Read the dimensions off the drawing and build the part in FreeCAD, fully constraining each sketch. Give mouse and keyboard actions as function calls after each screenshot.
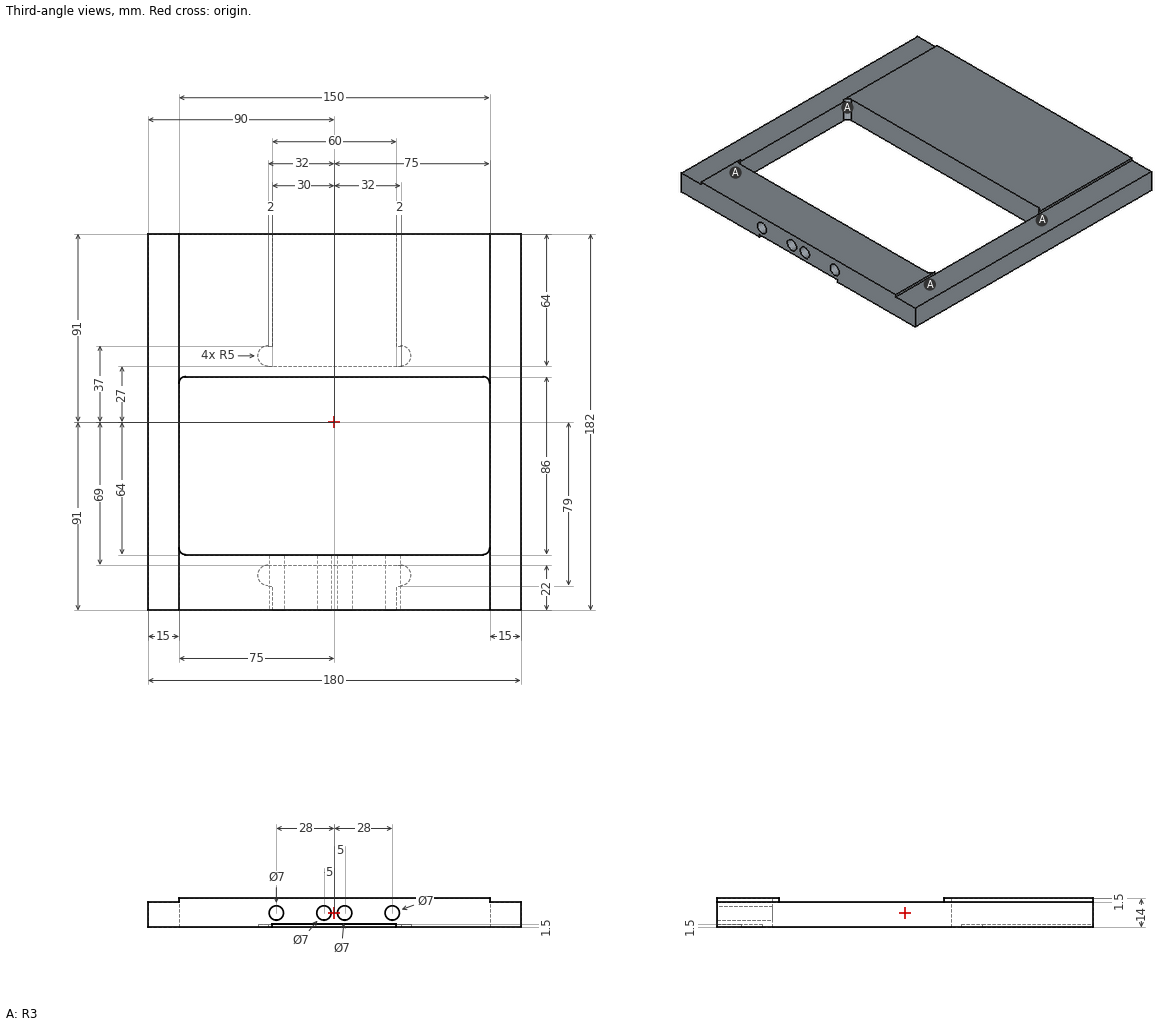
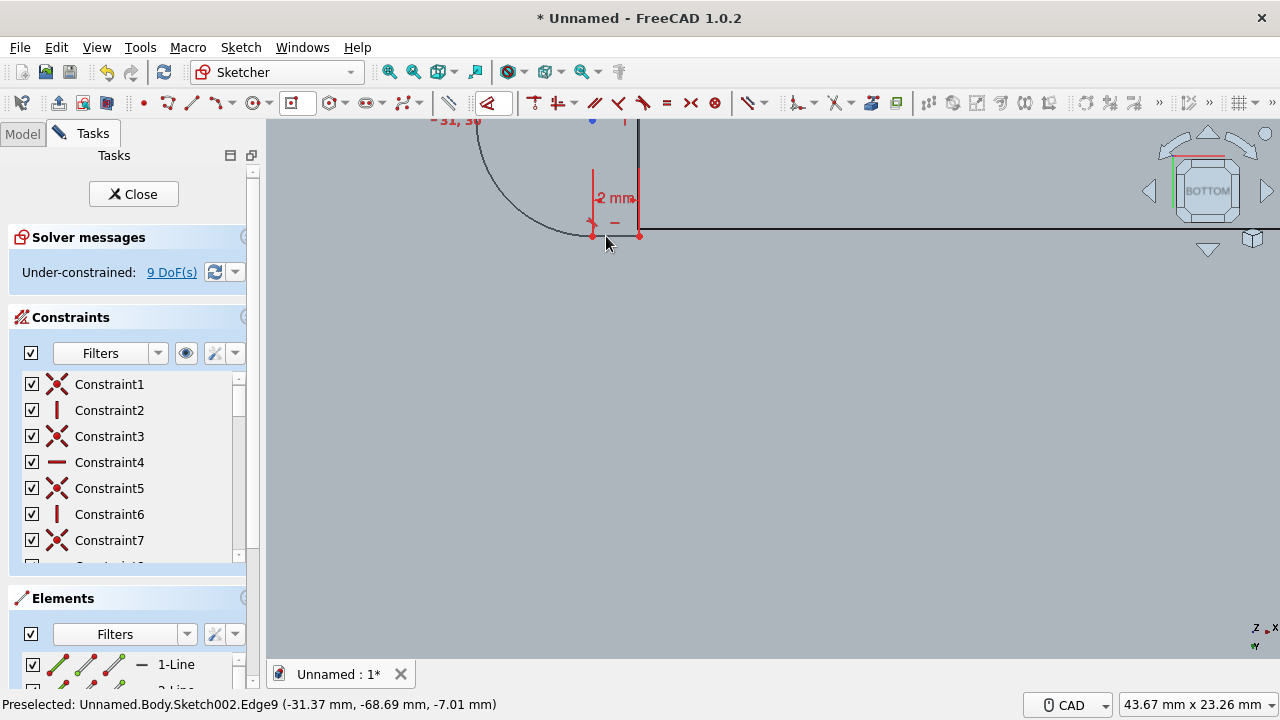
scroll(606, 240, down, 10)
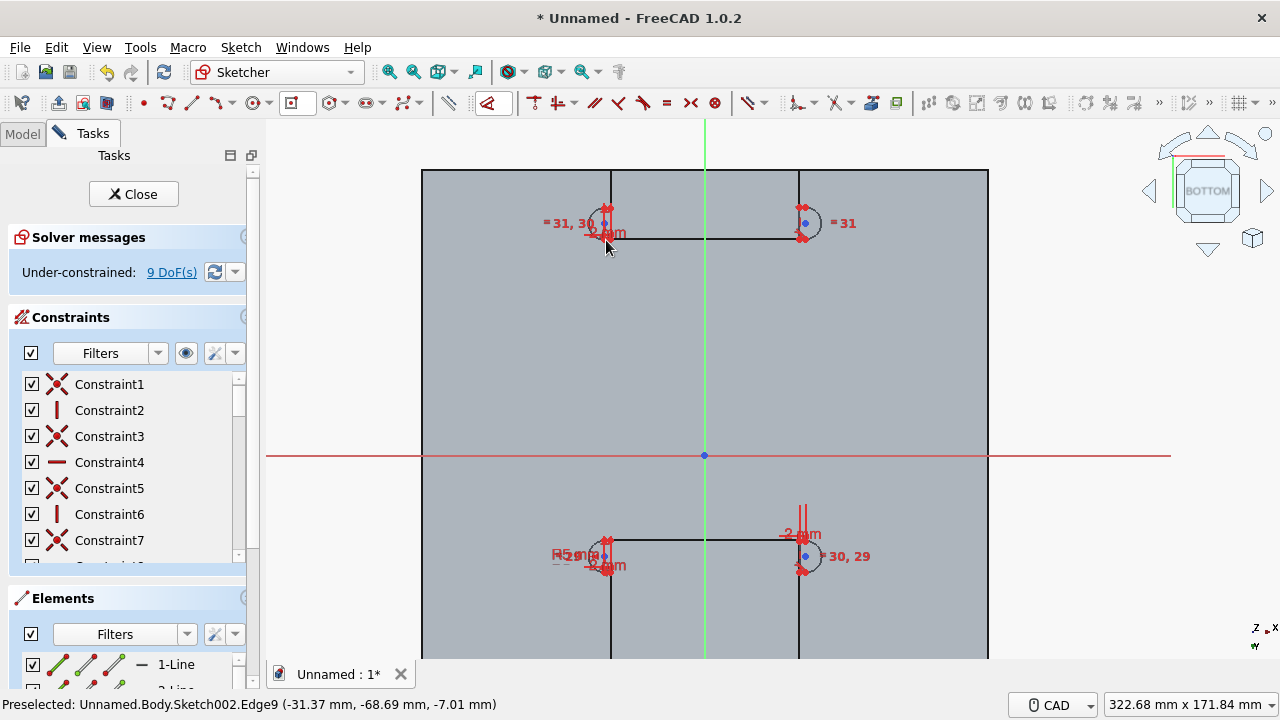
scroll(804, 208, up, 10)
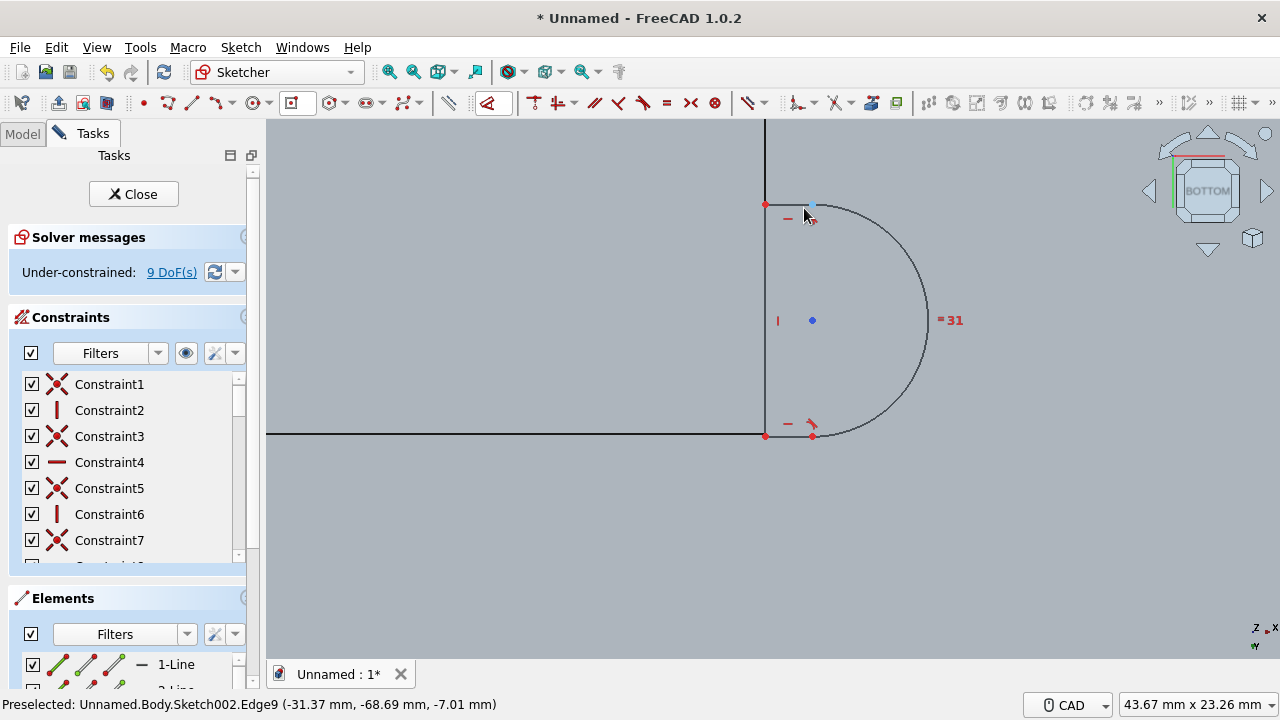
click(798, 205)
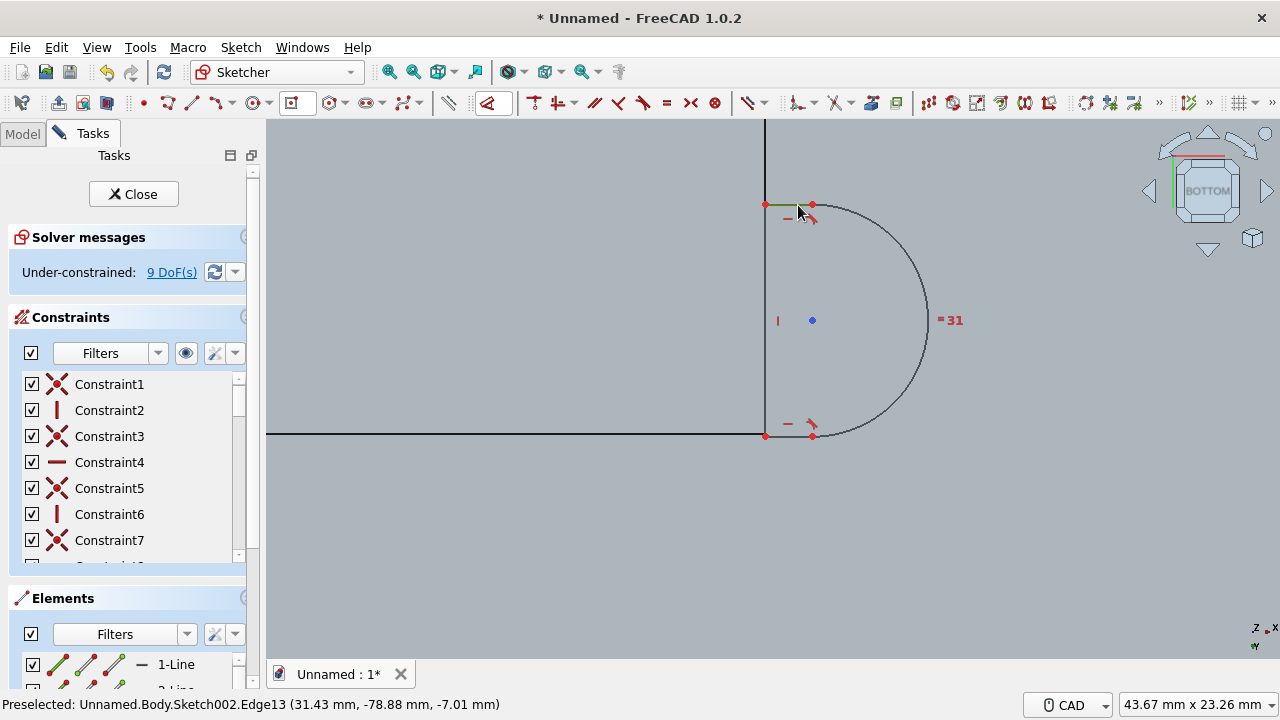
key(l)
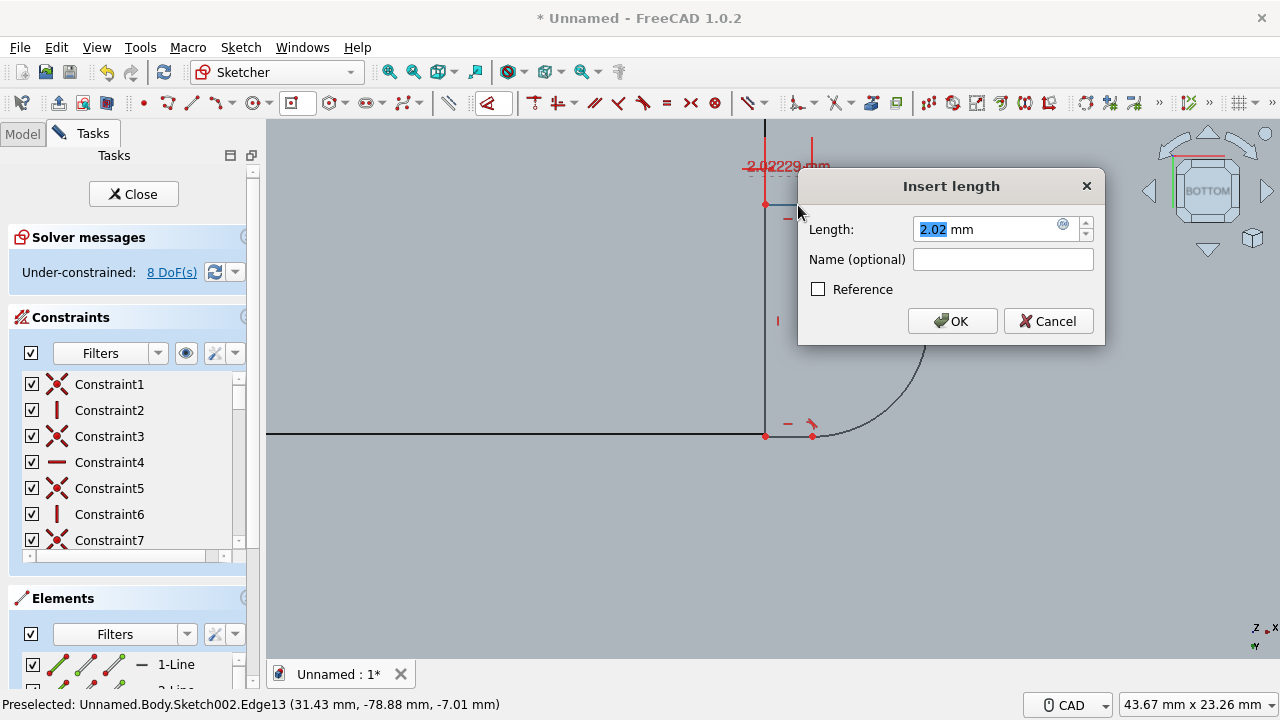
text(2)
key(Return)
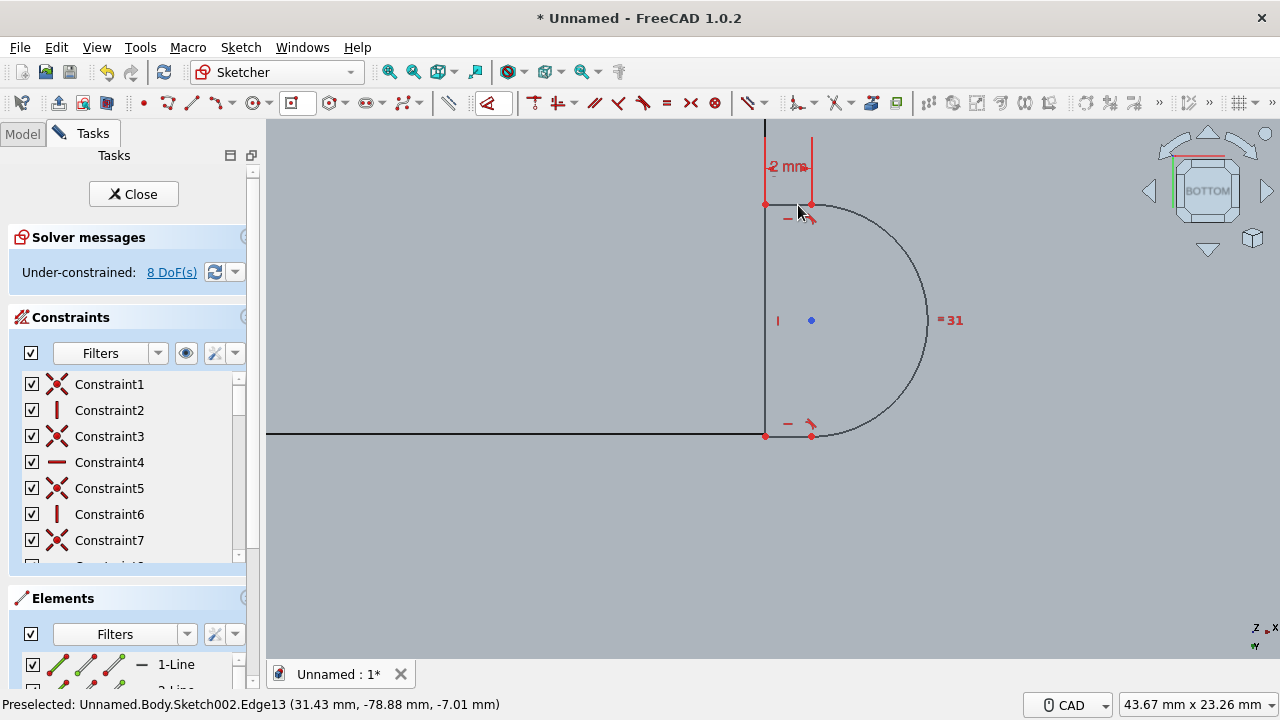
scroll(804, 208, down, 10)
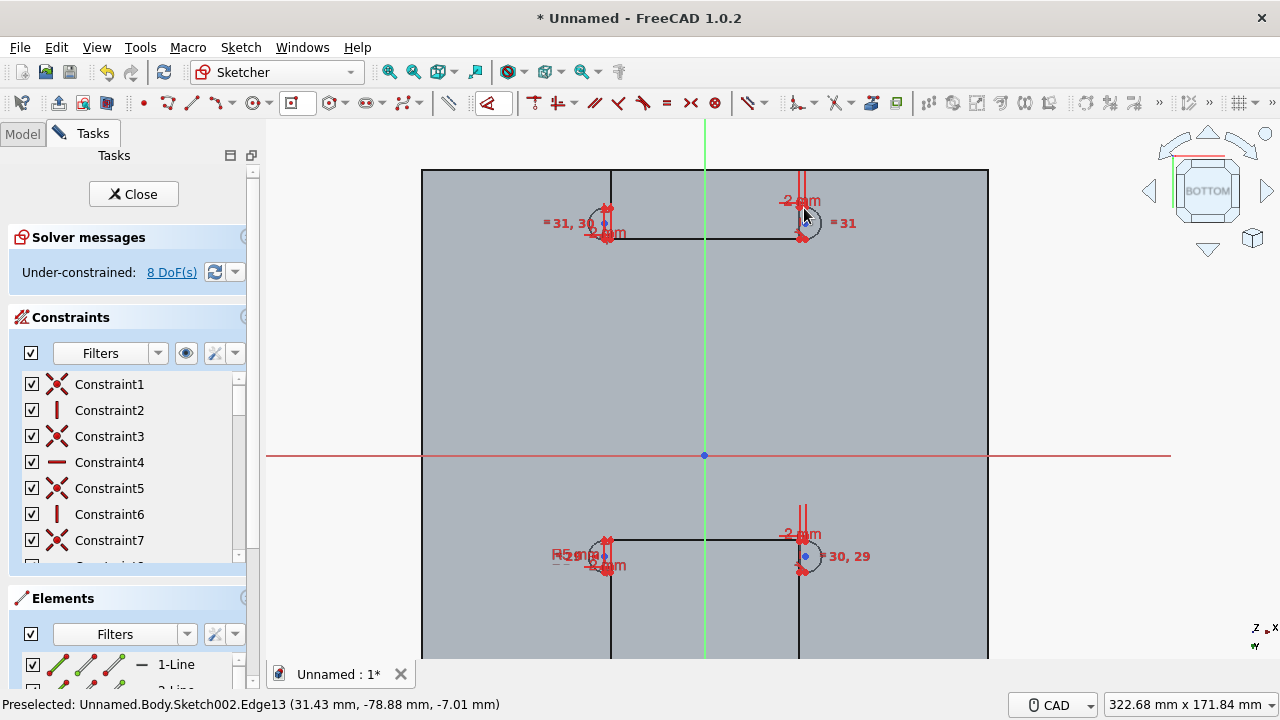
scroll(604, 572, up, 4)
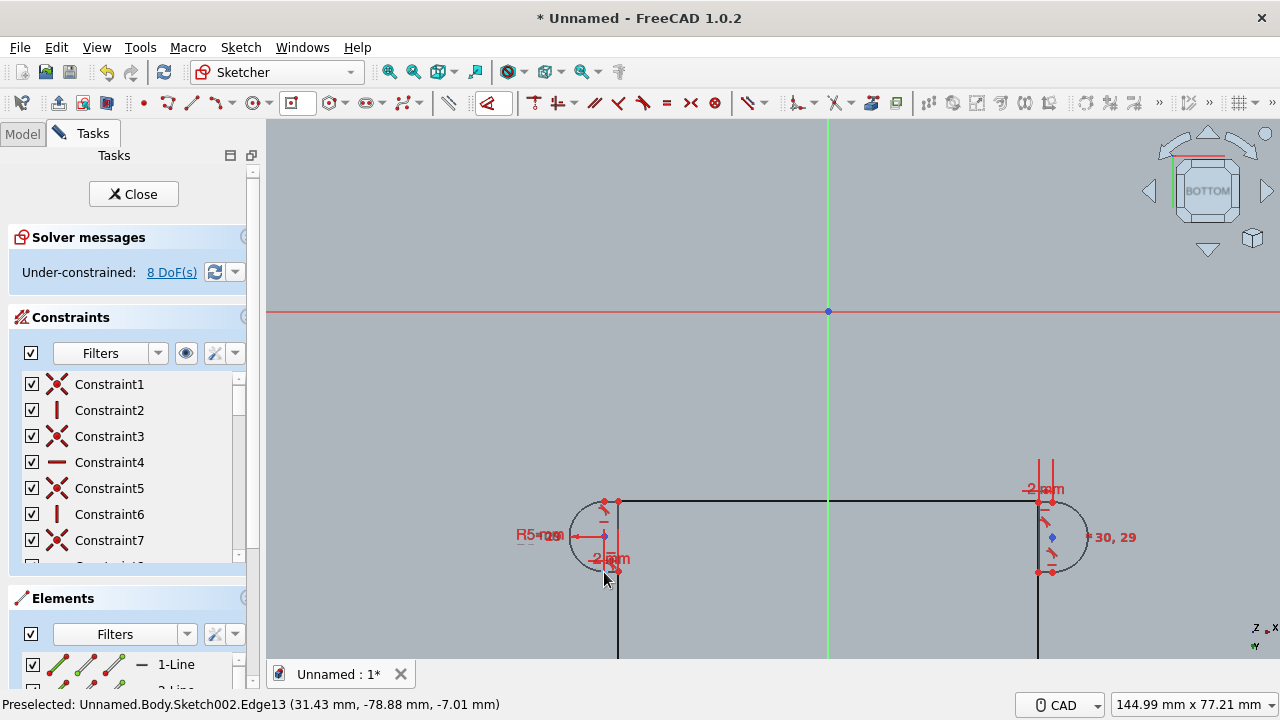
click(604, 572)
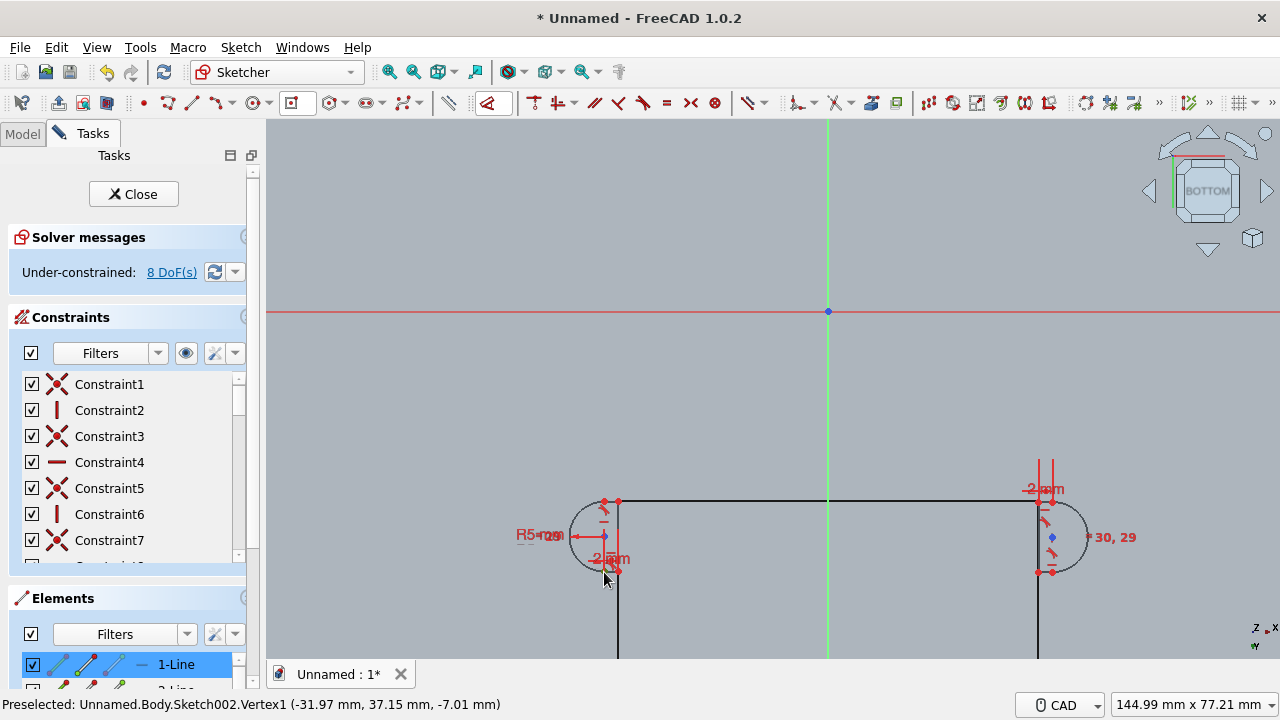
key(l)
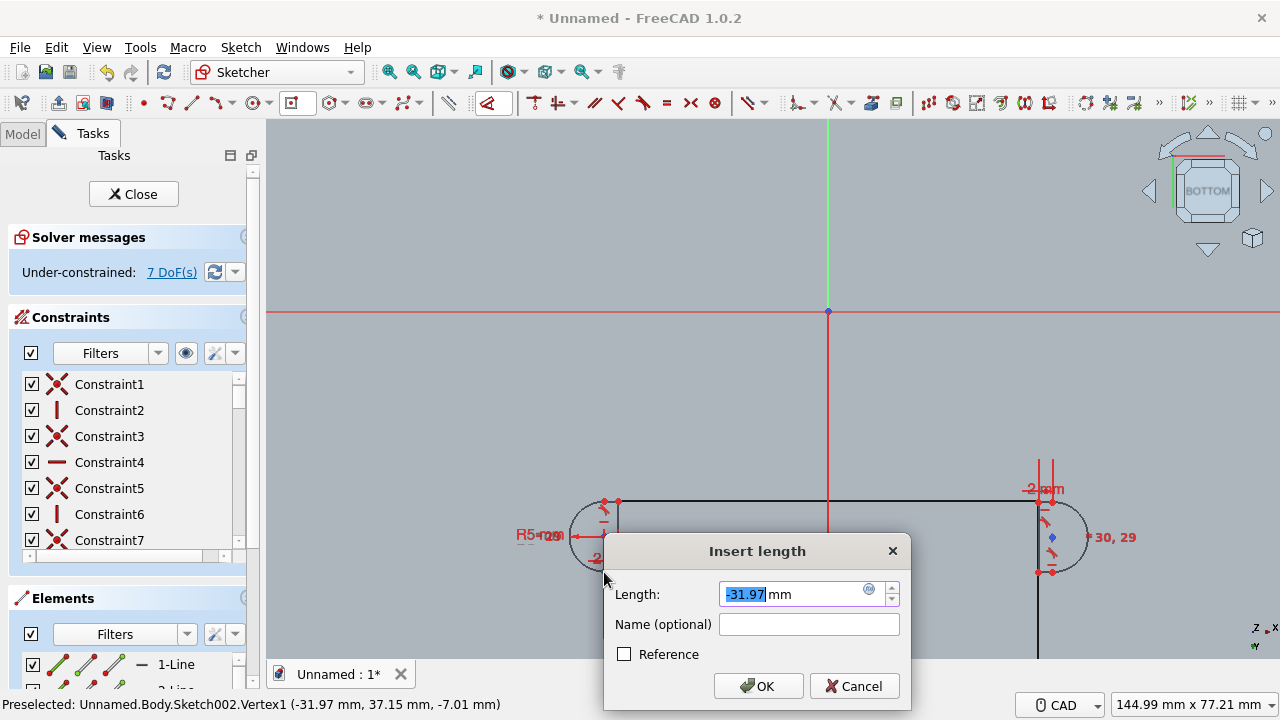
text(-32)
key(Return)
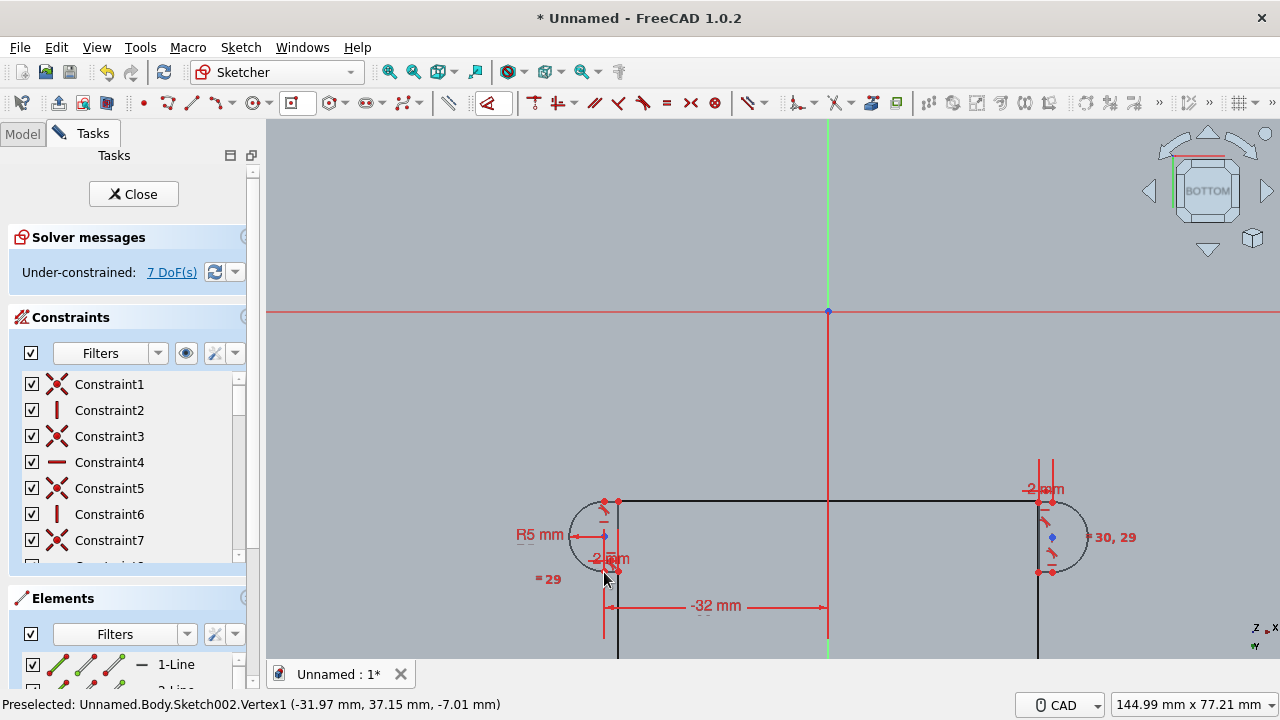
click(604, 572)